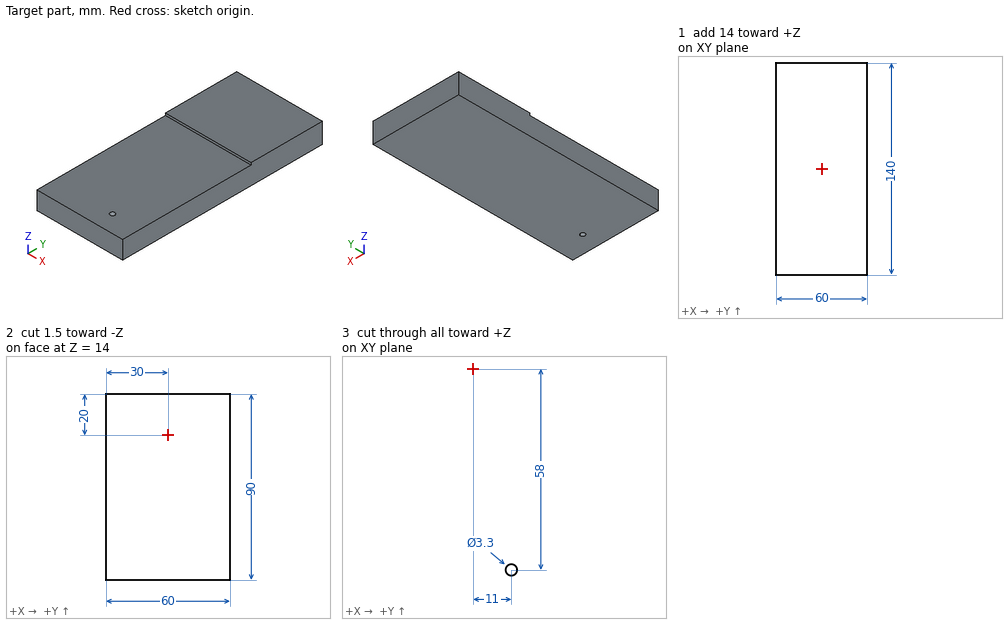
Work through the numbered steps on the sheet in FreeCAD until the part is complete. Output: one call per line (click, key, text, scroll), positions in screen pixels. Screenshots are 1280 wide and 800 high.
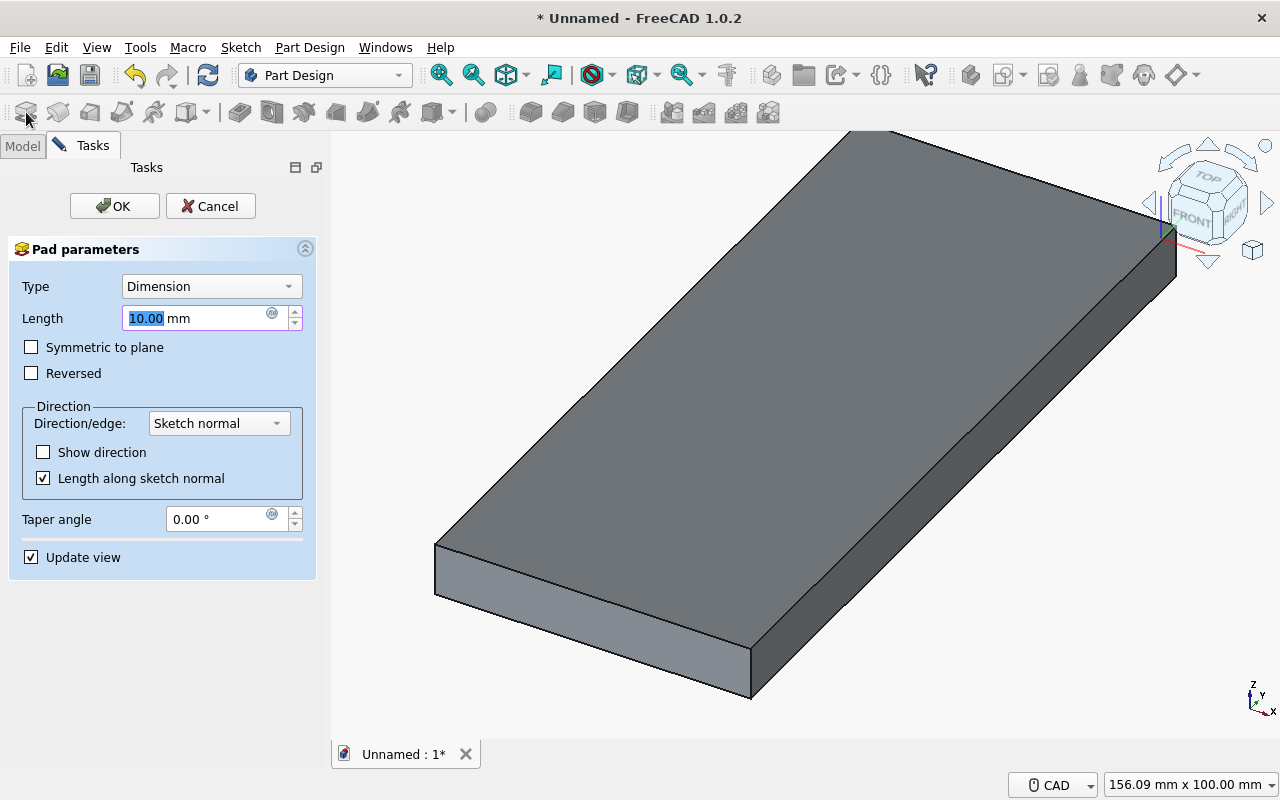
text(14)
key(Tab)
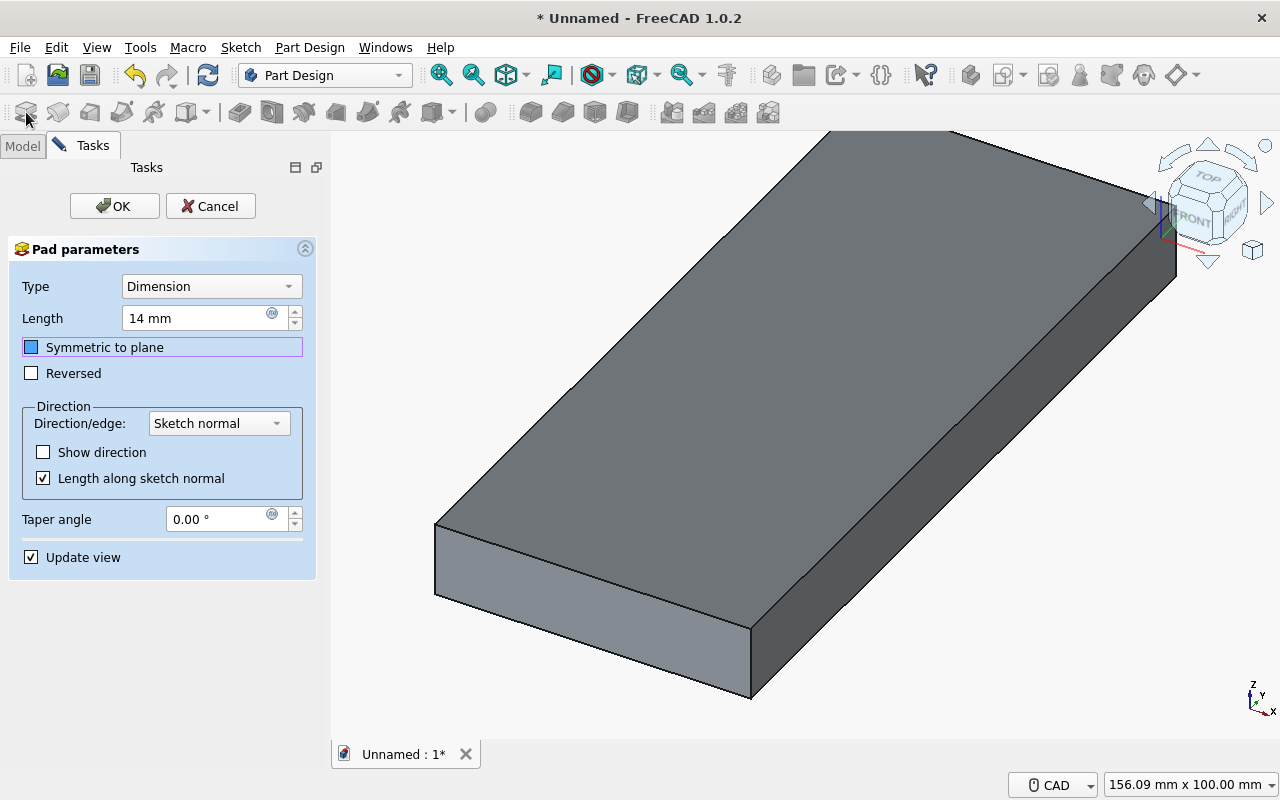
click(115, 206)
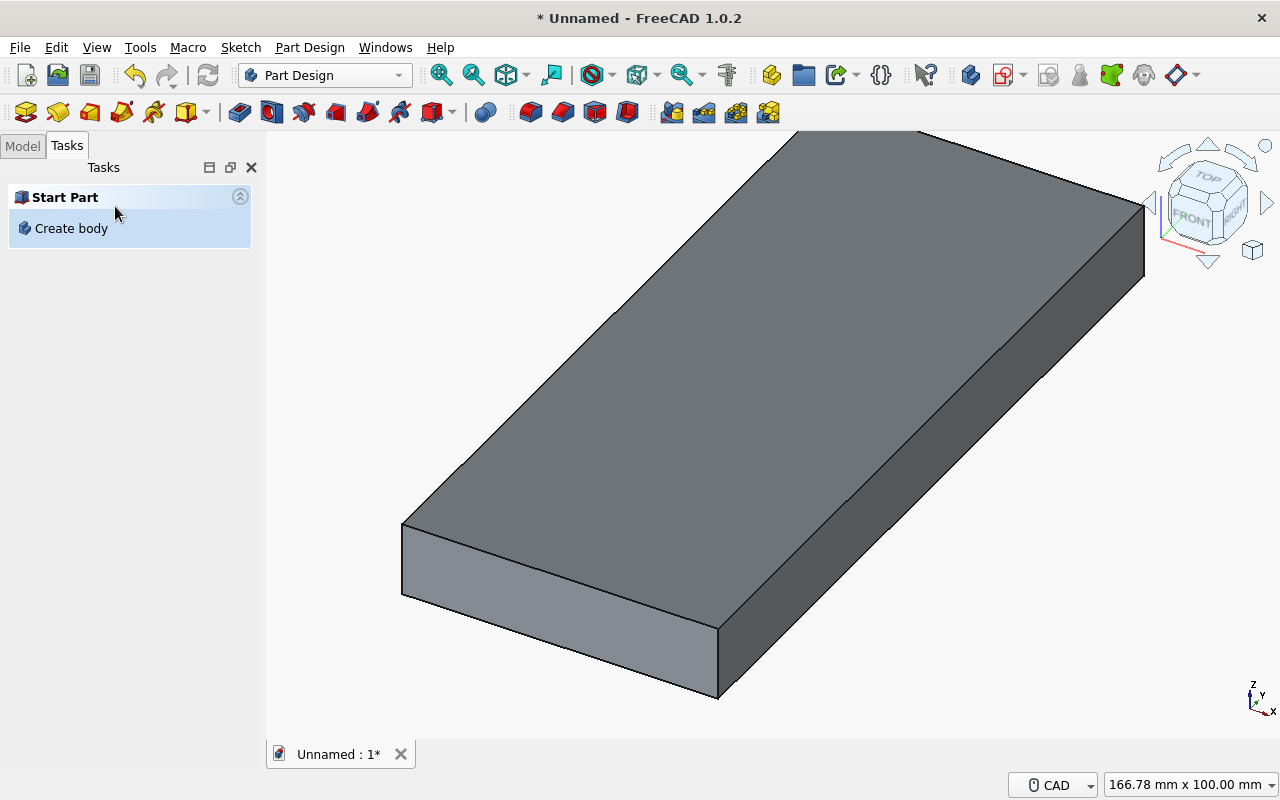
click(442, 76)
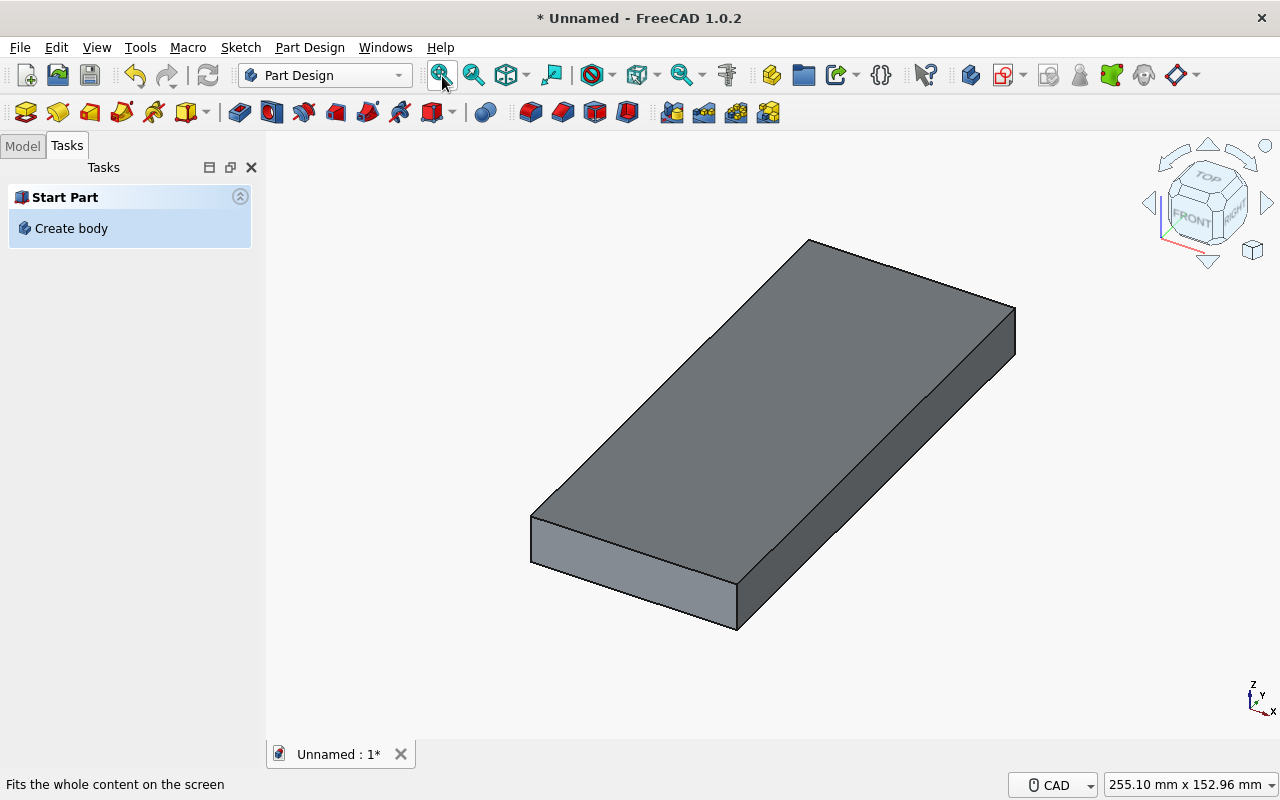
click(852, 332)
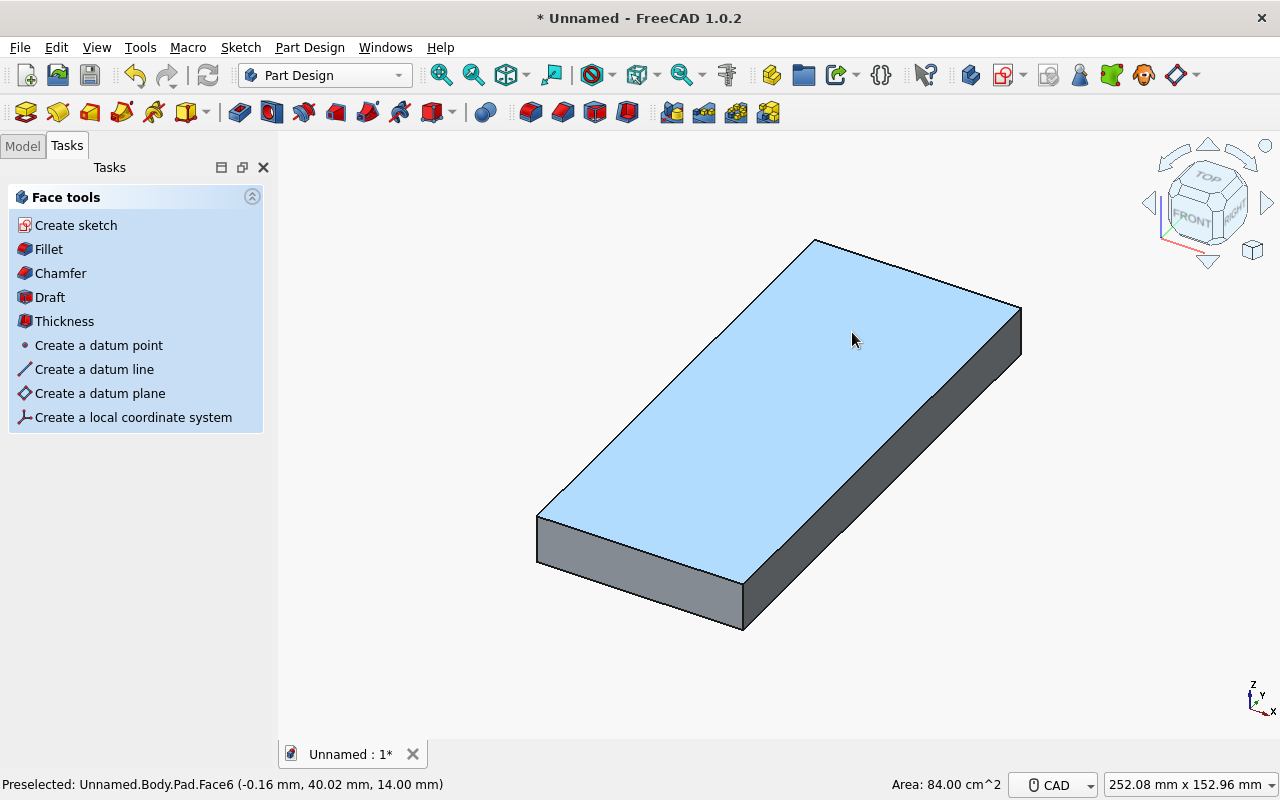
click(1004, 76)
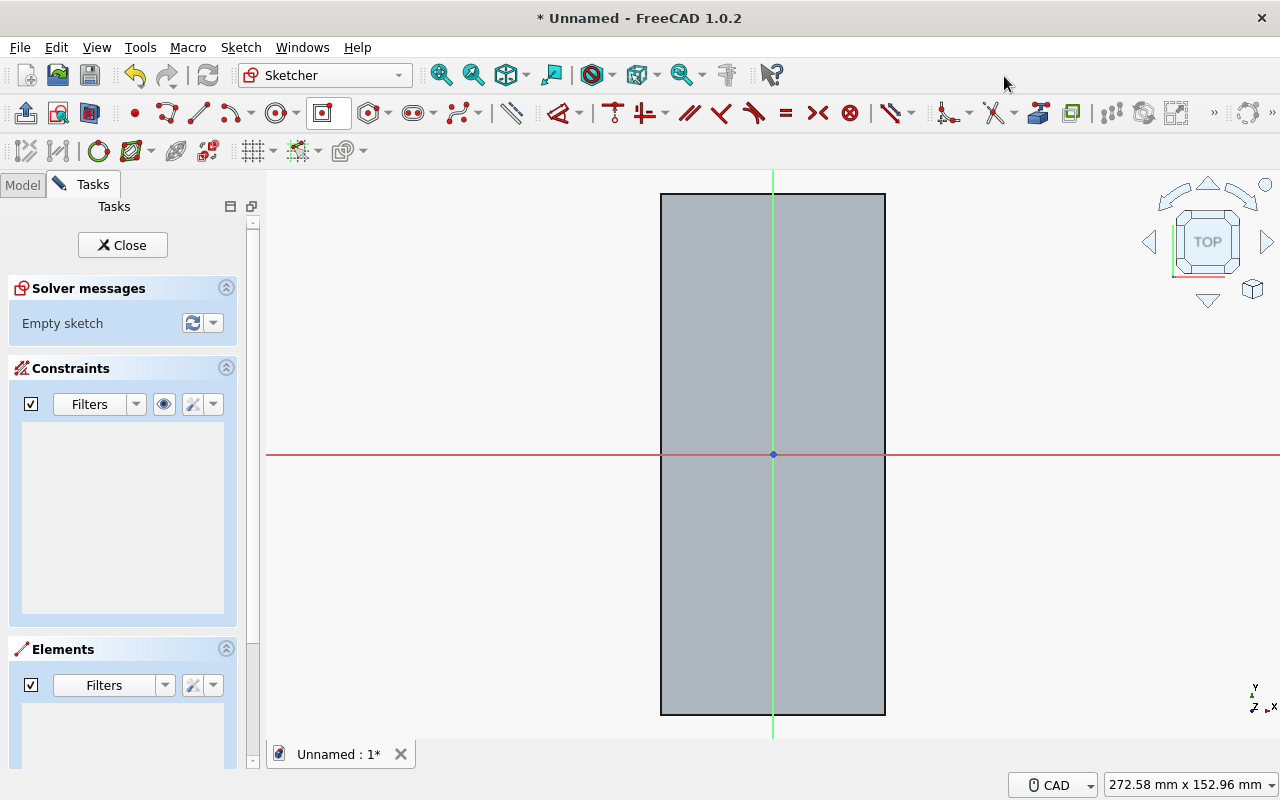
scroll(395, 198, down, 1)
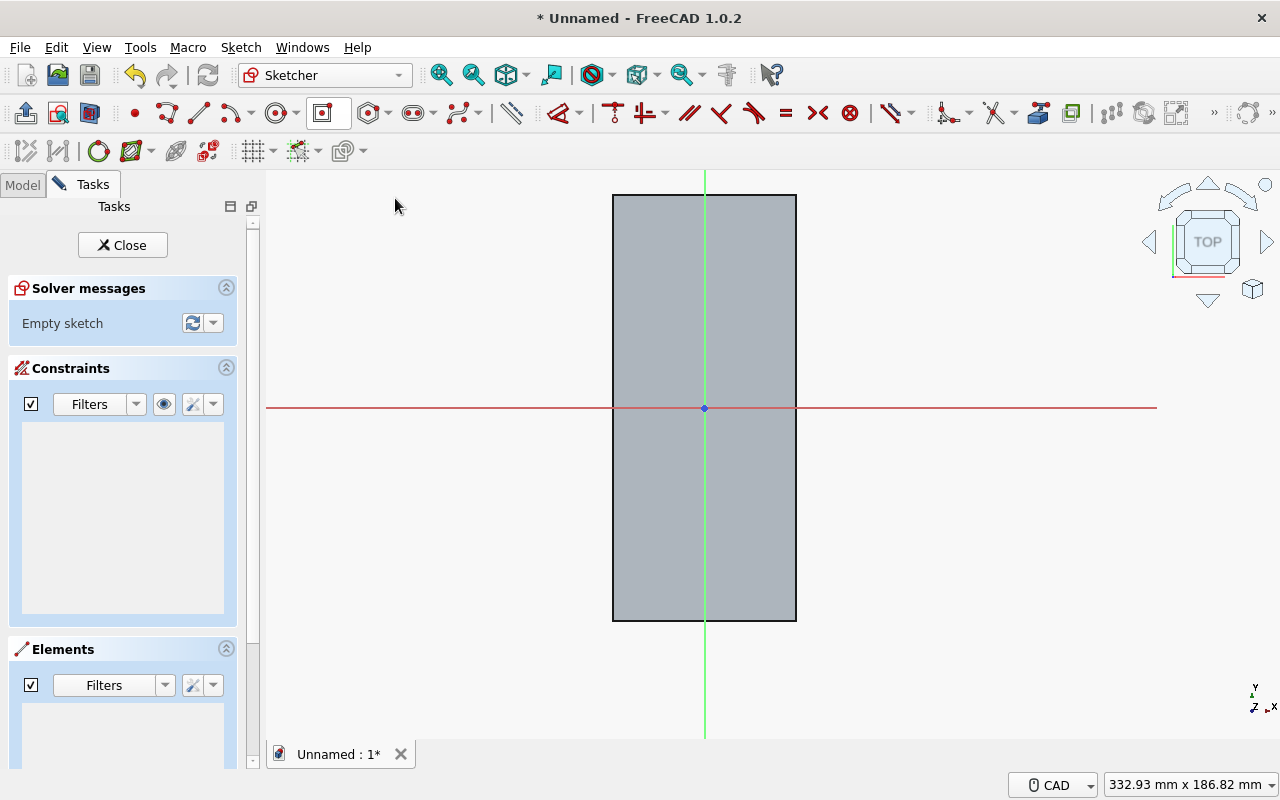
click(346, 114)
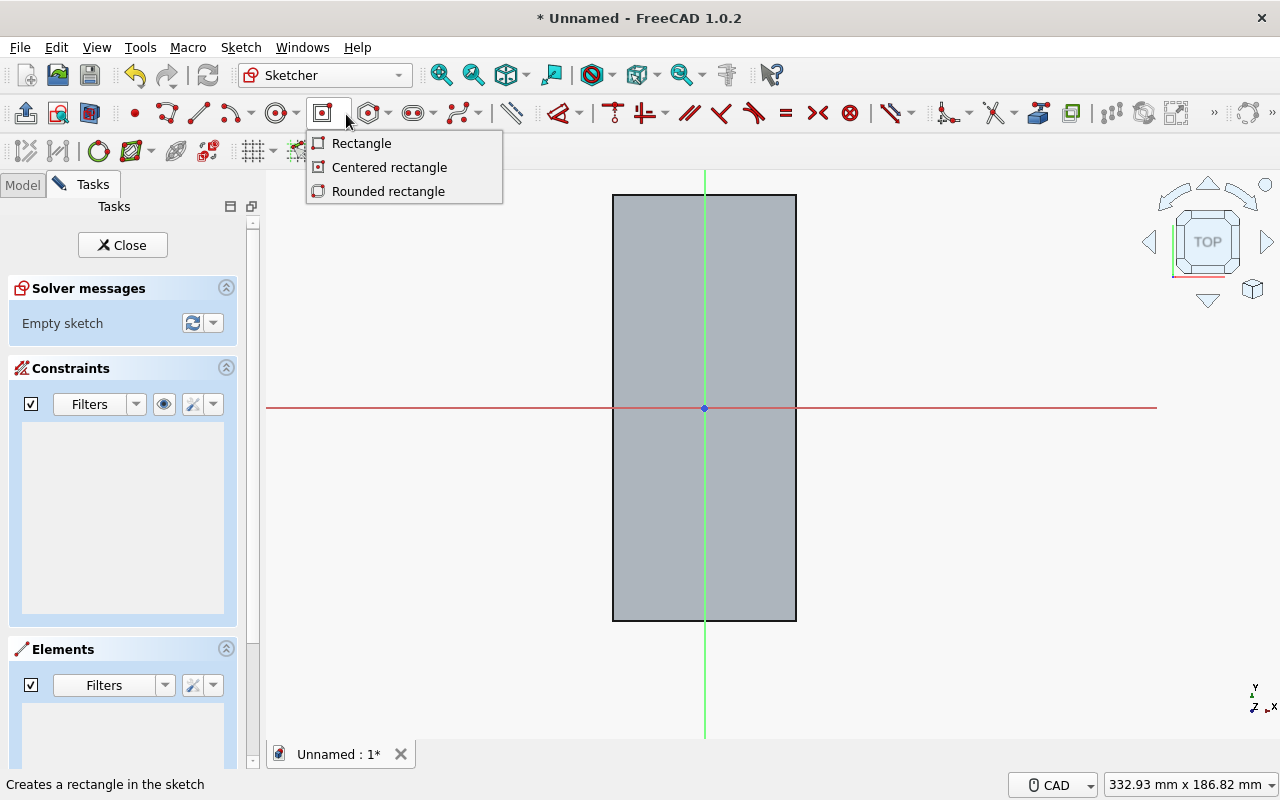
click(404, 143)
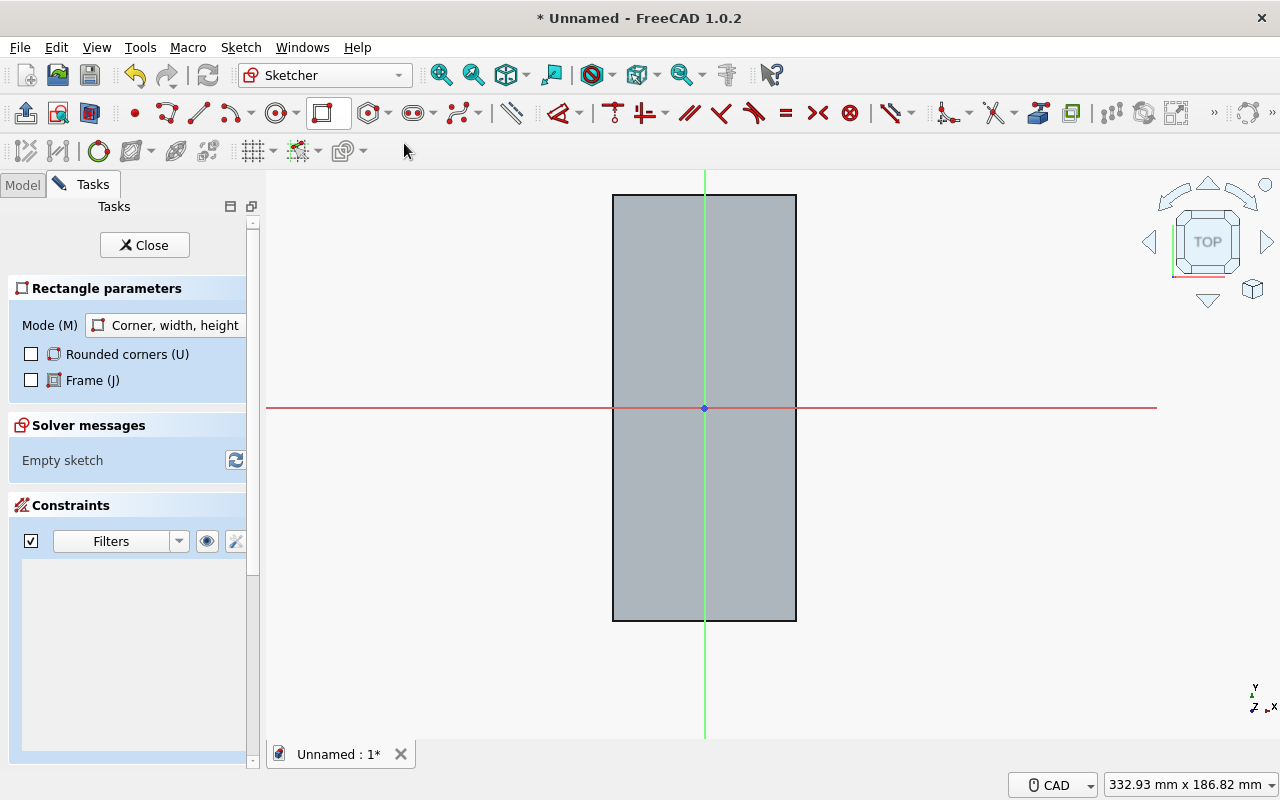
click(613, 347)
move(796, 621)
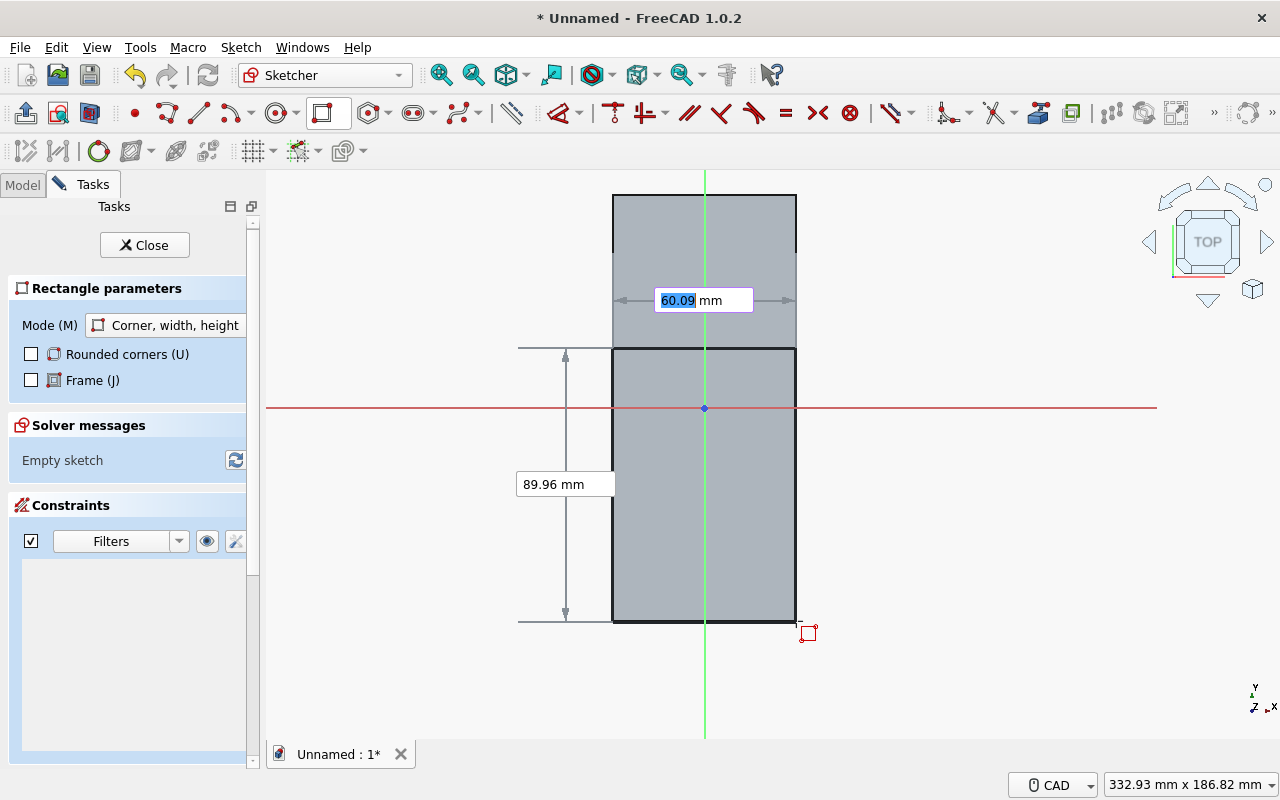
text(60)
key(Tab)
text(90)
key(Return)
key(Escape)